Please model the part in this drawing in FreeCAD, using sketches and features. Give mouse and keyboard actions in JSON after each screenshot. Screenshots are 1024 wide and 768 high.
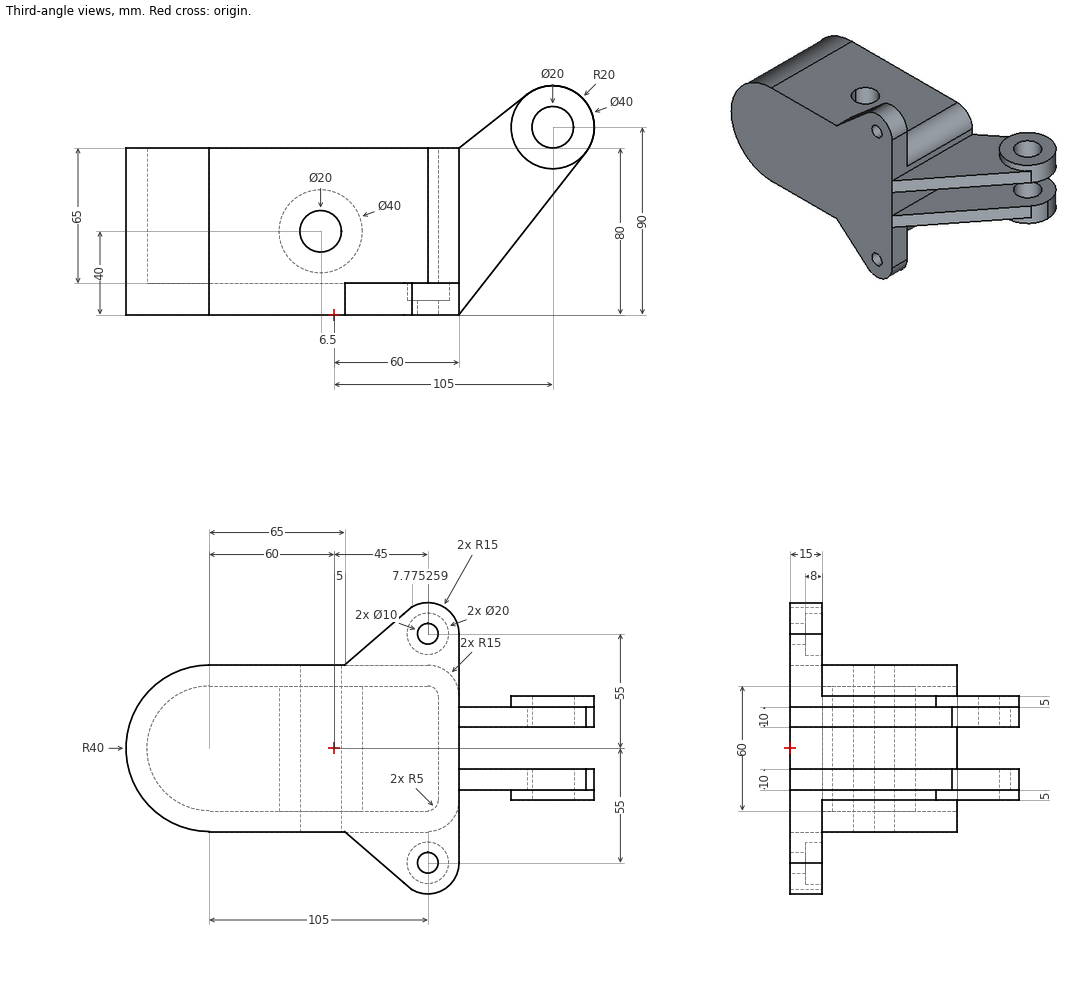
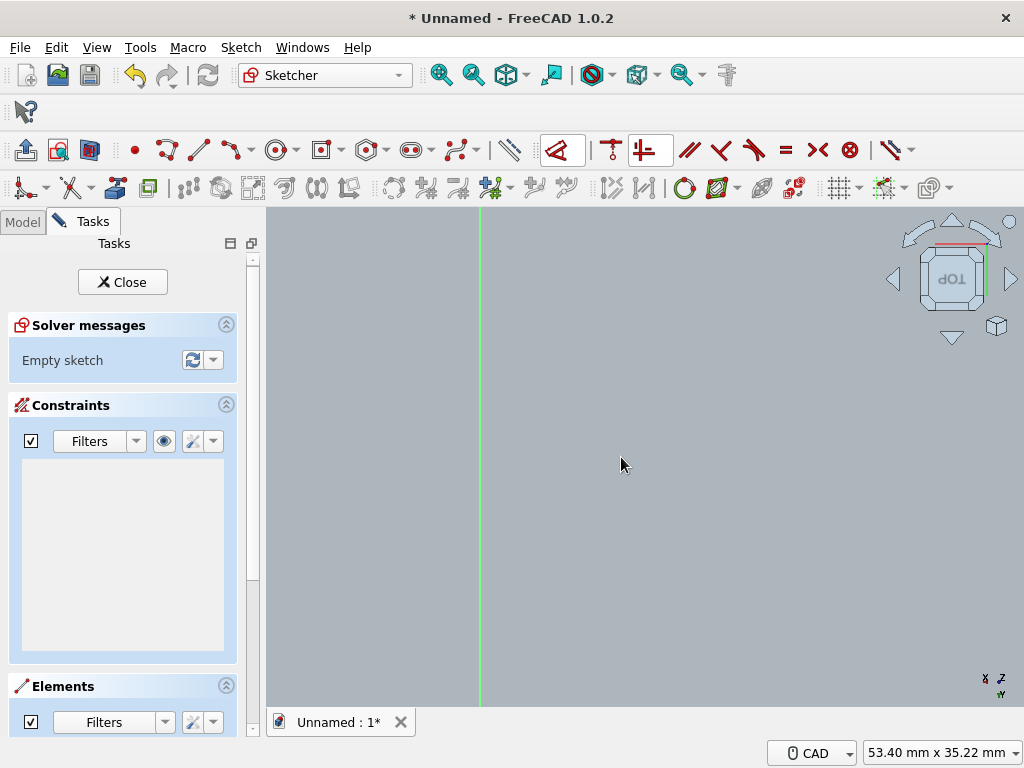
{"action": "left_click", "coordinate": [276, 150]}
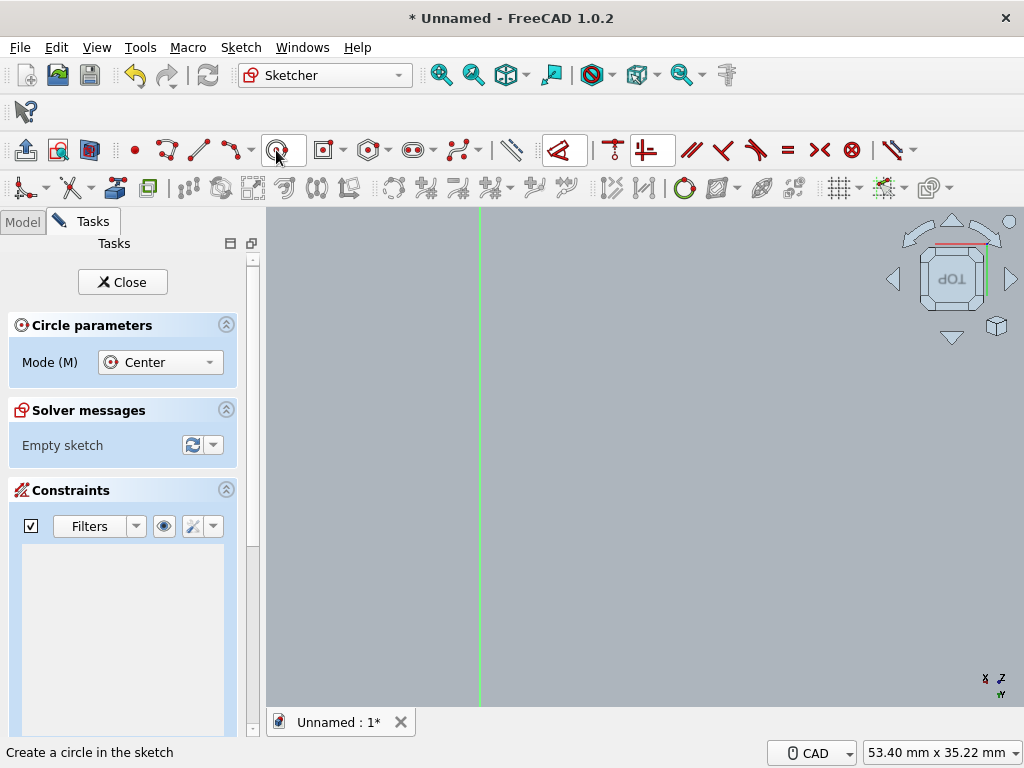
{"action": "left_click", "coordinate": [572, 454]}
{"action": "left_click", "coordinate": [673, 354]}
{"action": "key", "text": "Escape"}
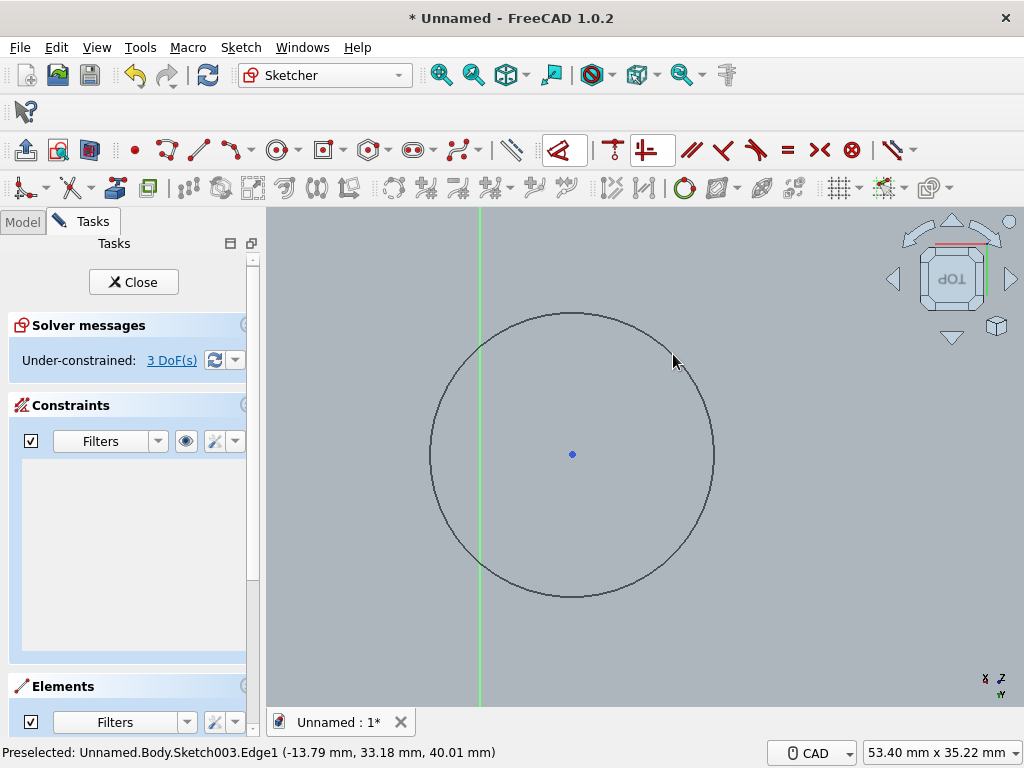
{"action": "left_click", "coordinate": [672, 354]}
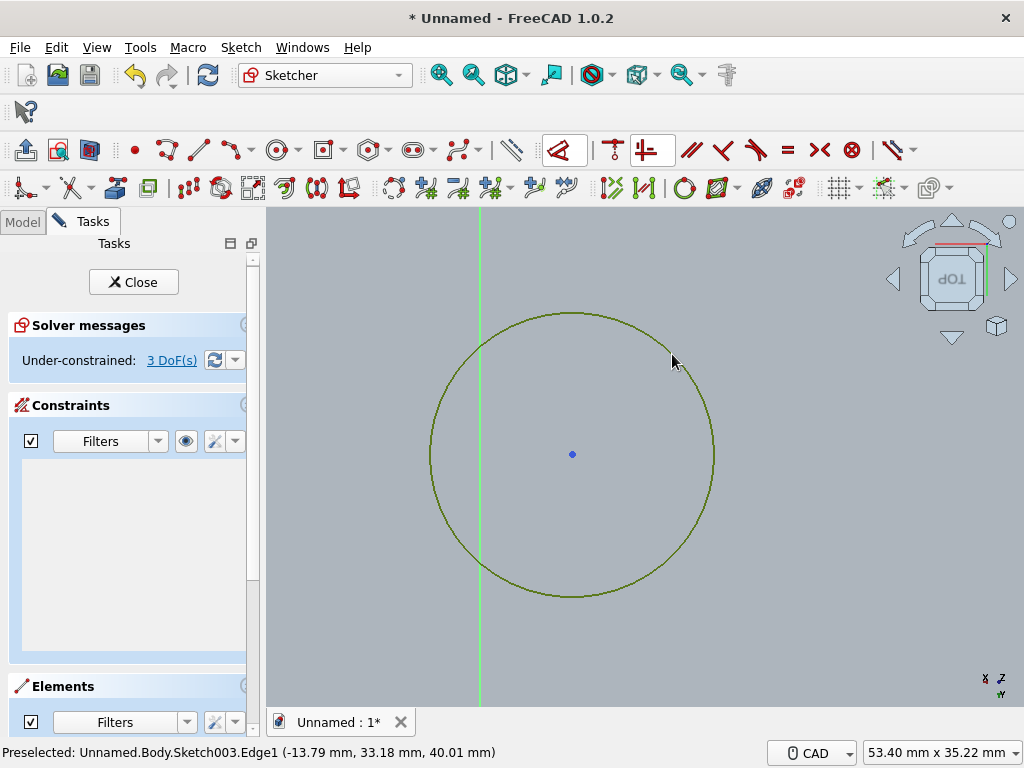
{"action": "left_click", "coordinate": [582, 150]}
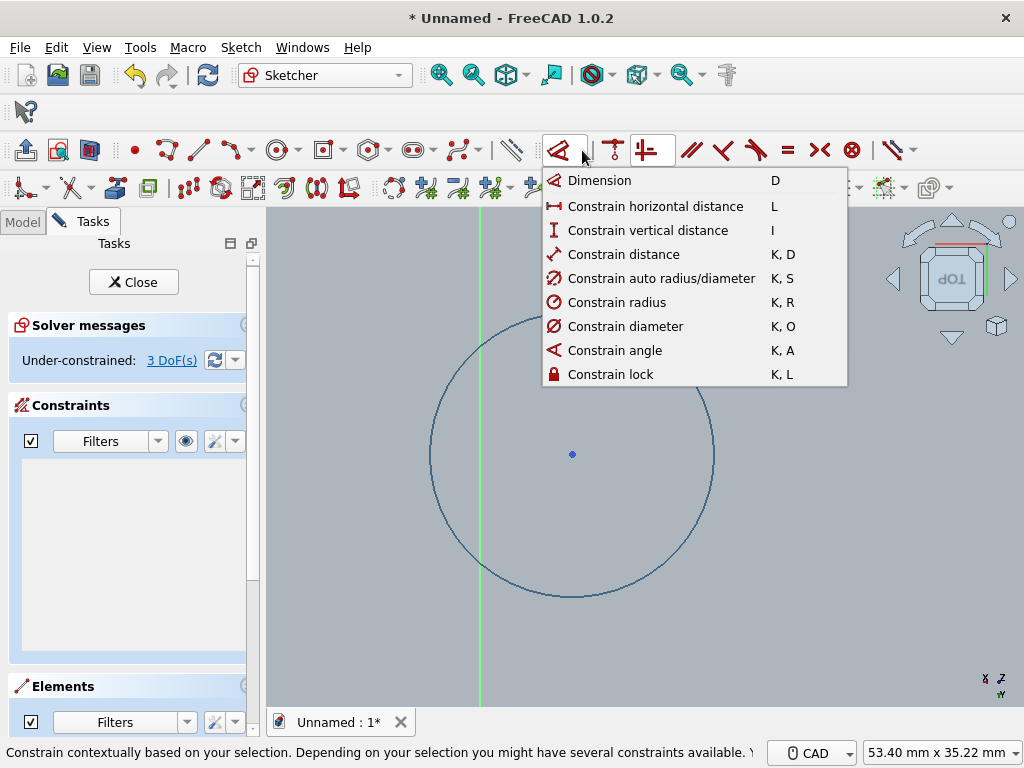
{"action": "left_click", "coordinate": [695, 326]}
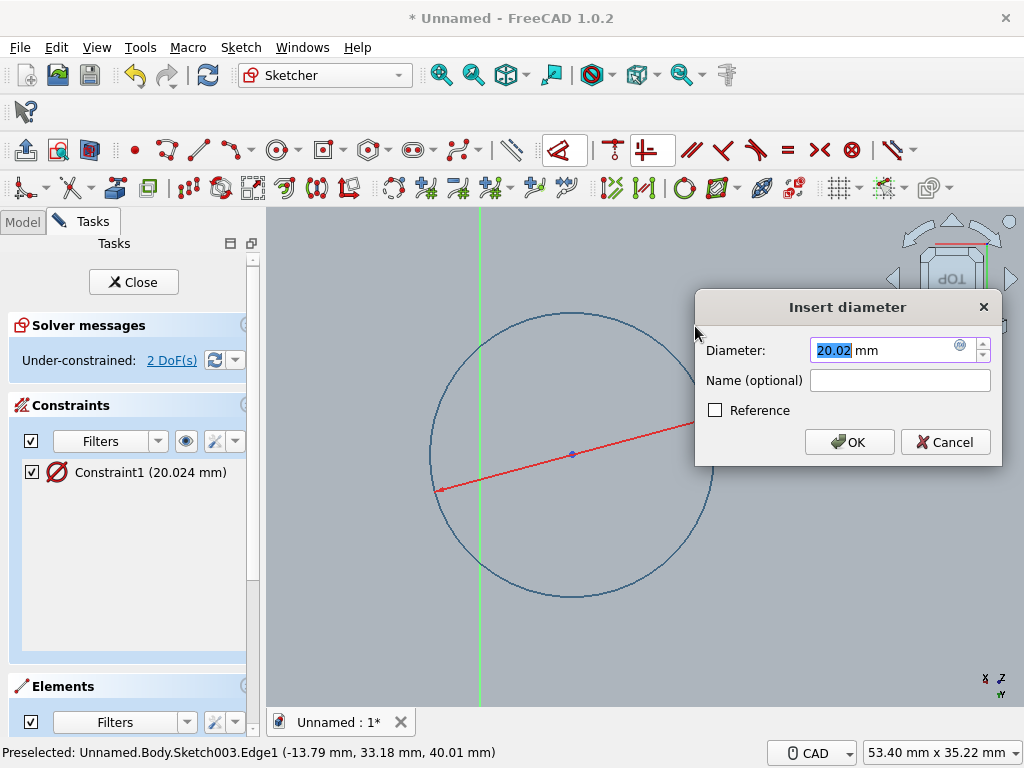
{"action": "type", "text": "20"}
{"action": "key", "text": "Return"}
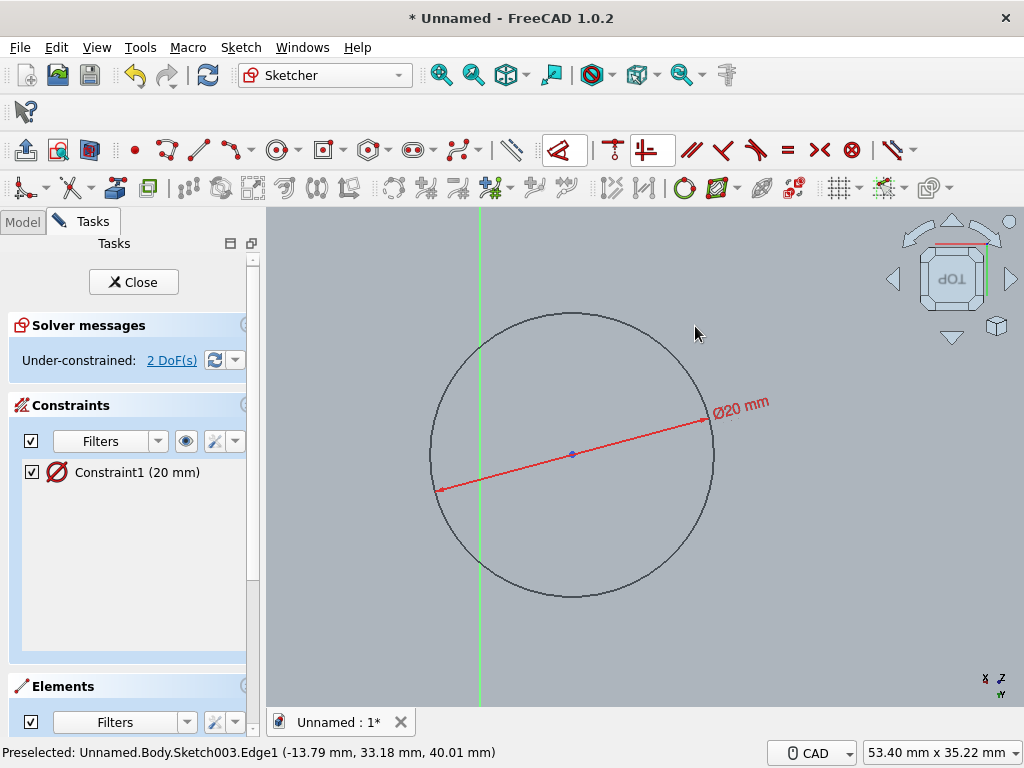
{"action": "left_click", "coordinate": [572, 455]}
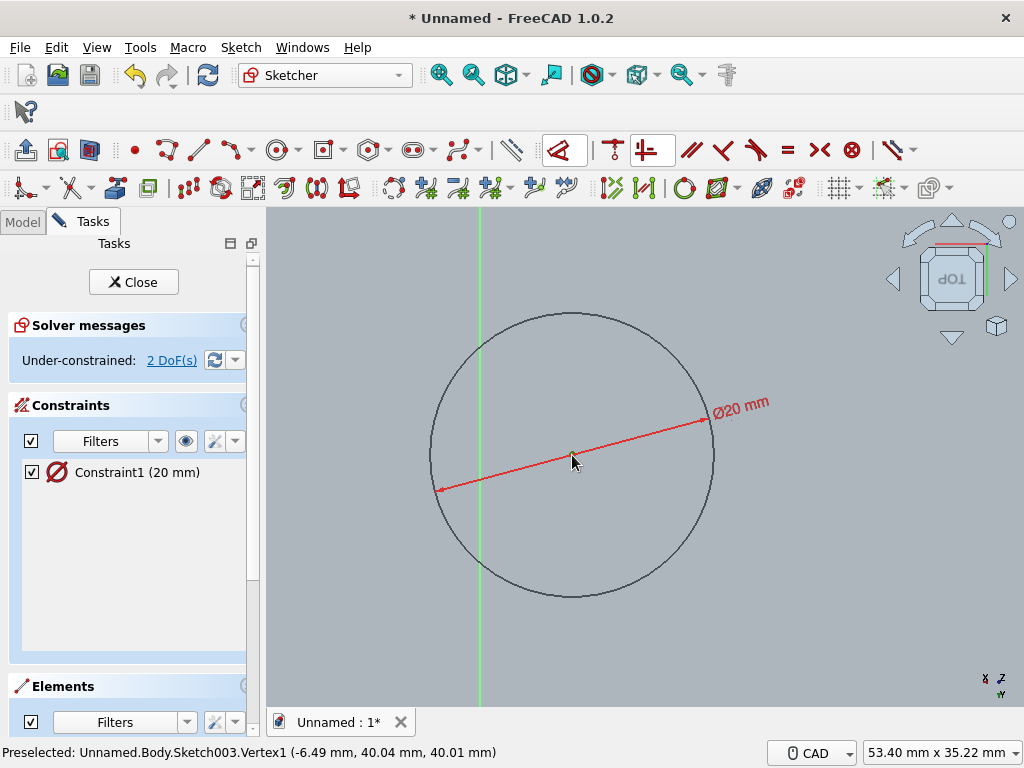
{"action": "left_click", "coordinate": [582, 150]}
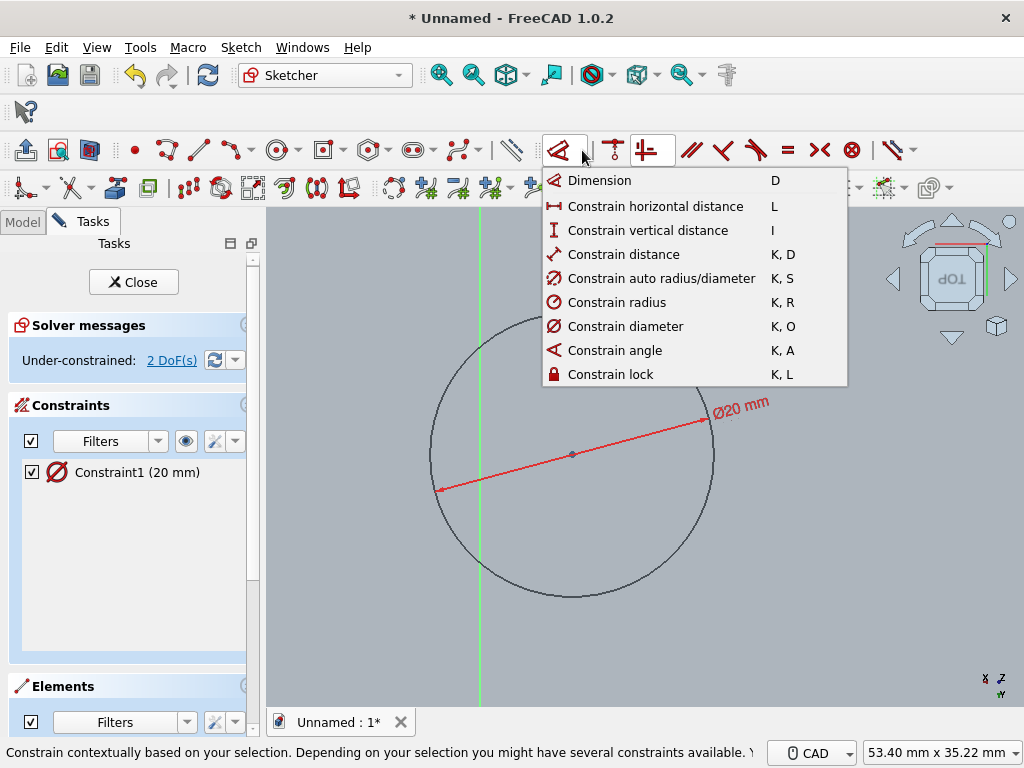
{"action": "left_click", "coordinate": [695, 230]}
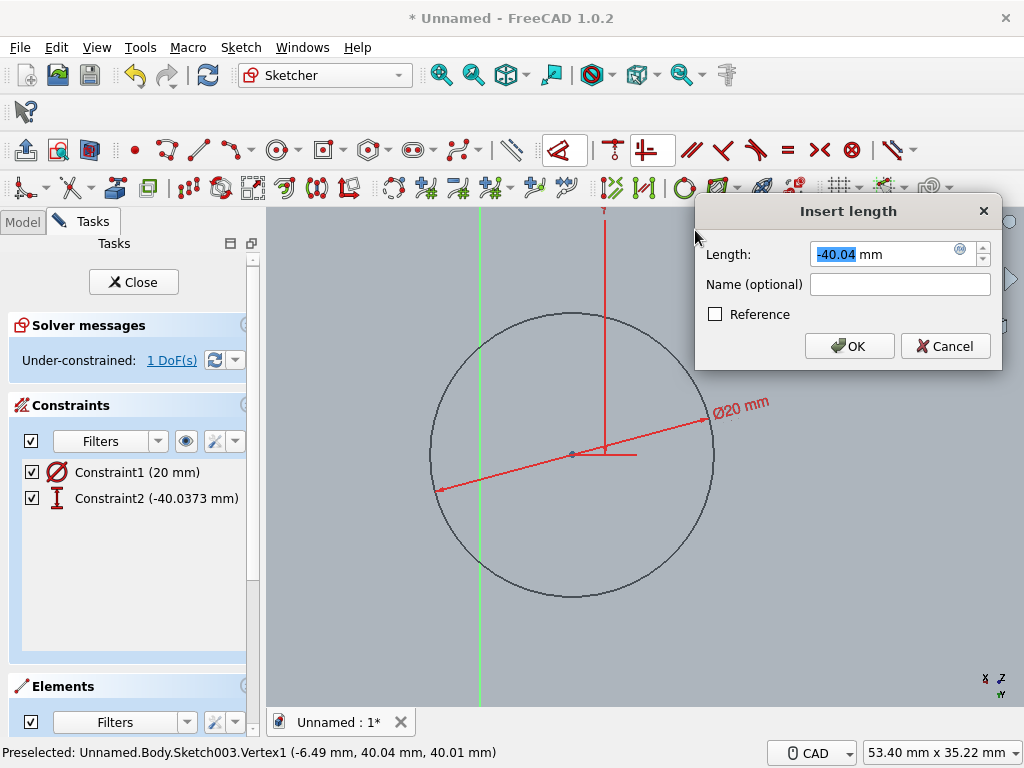
{"action": "type", "text": "-40"}
{"action": "key", "text": "Return"}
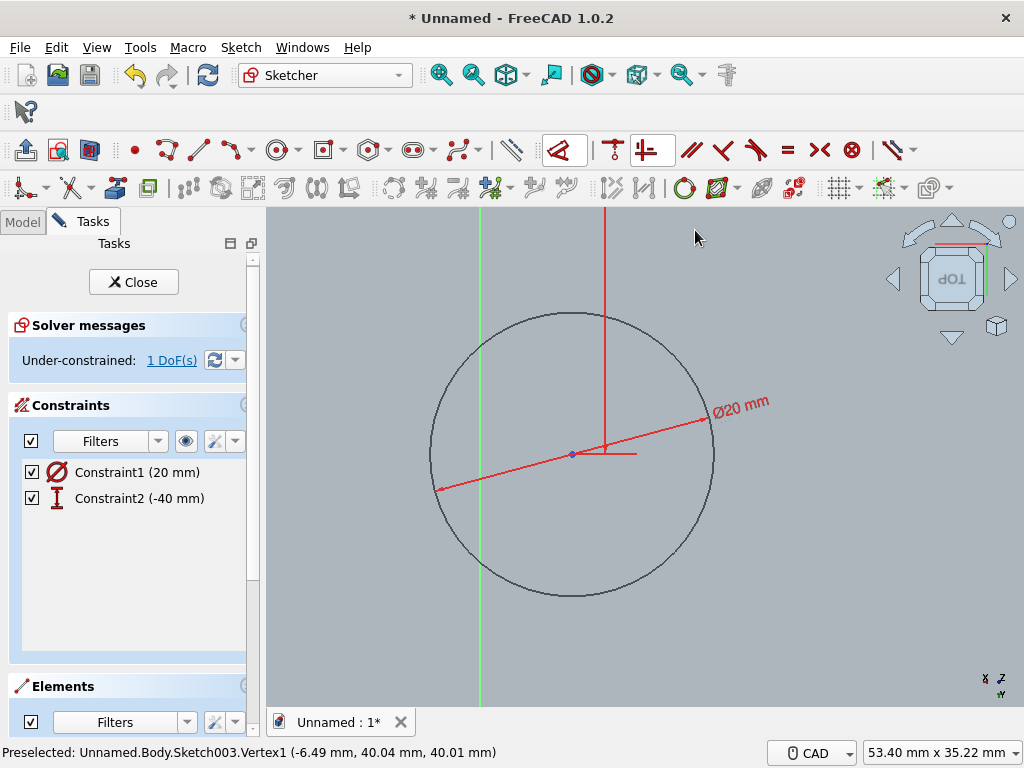
{"action": "left_click", "coordinate": [572, 454]}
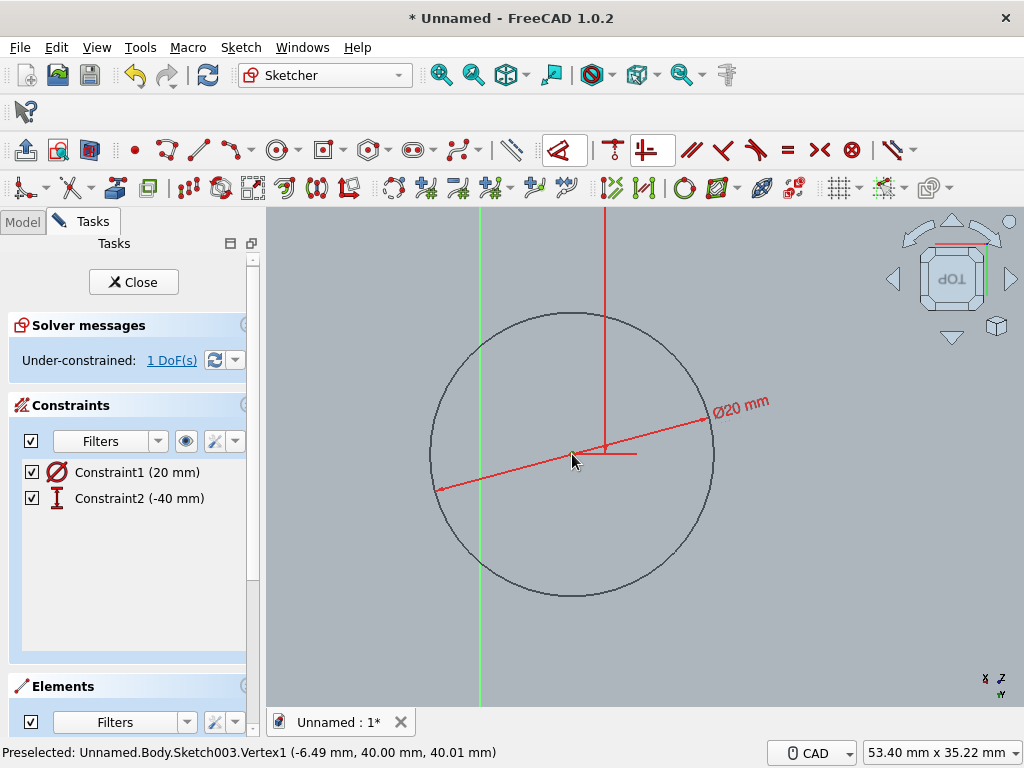
{"action": "key", "text": "l"}